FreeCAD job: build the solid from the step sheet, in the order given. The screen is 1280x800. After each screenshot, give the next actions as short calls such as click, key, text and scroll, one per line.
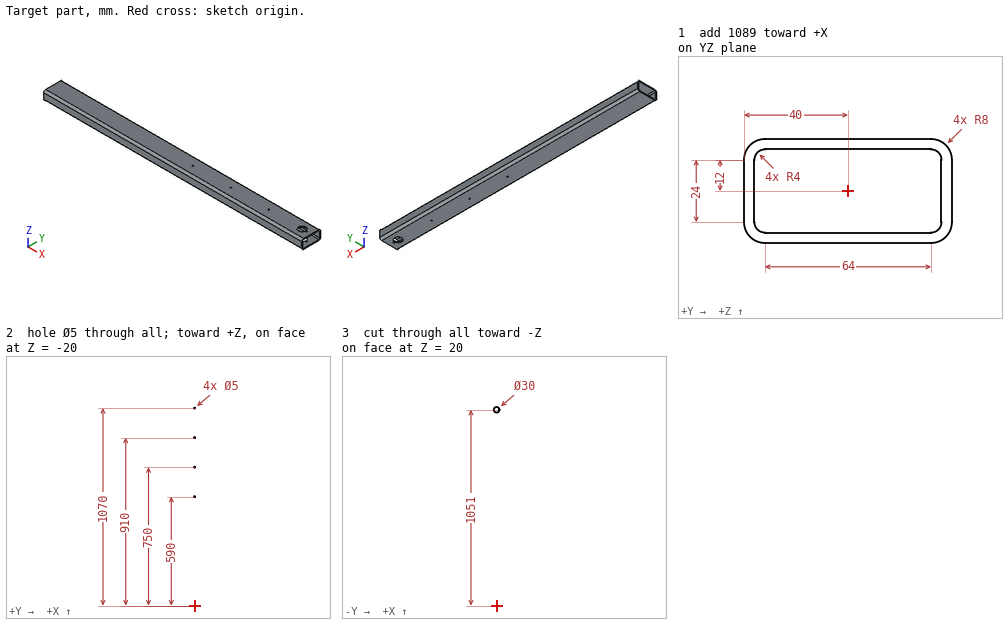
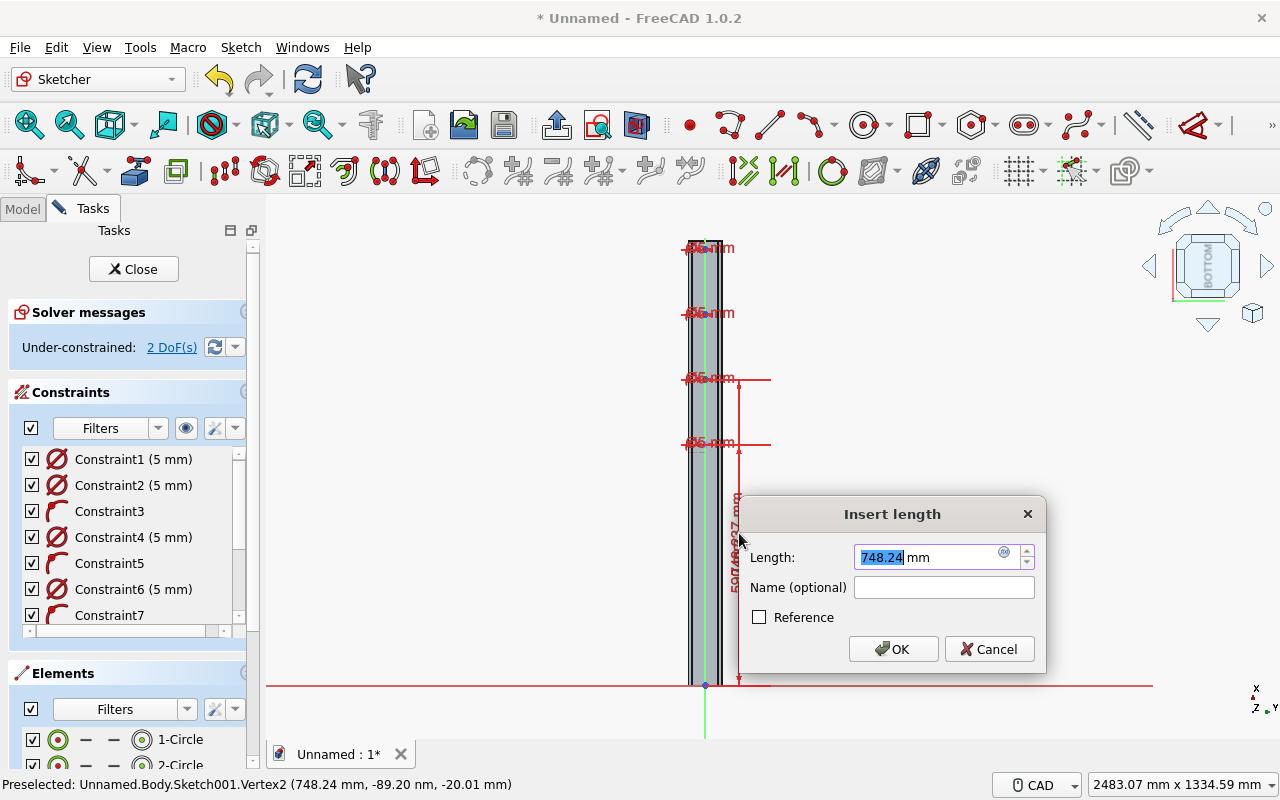
text(750)
key(Return)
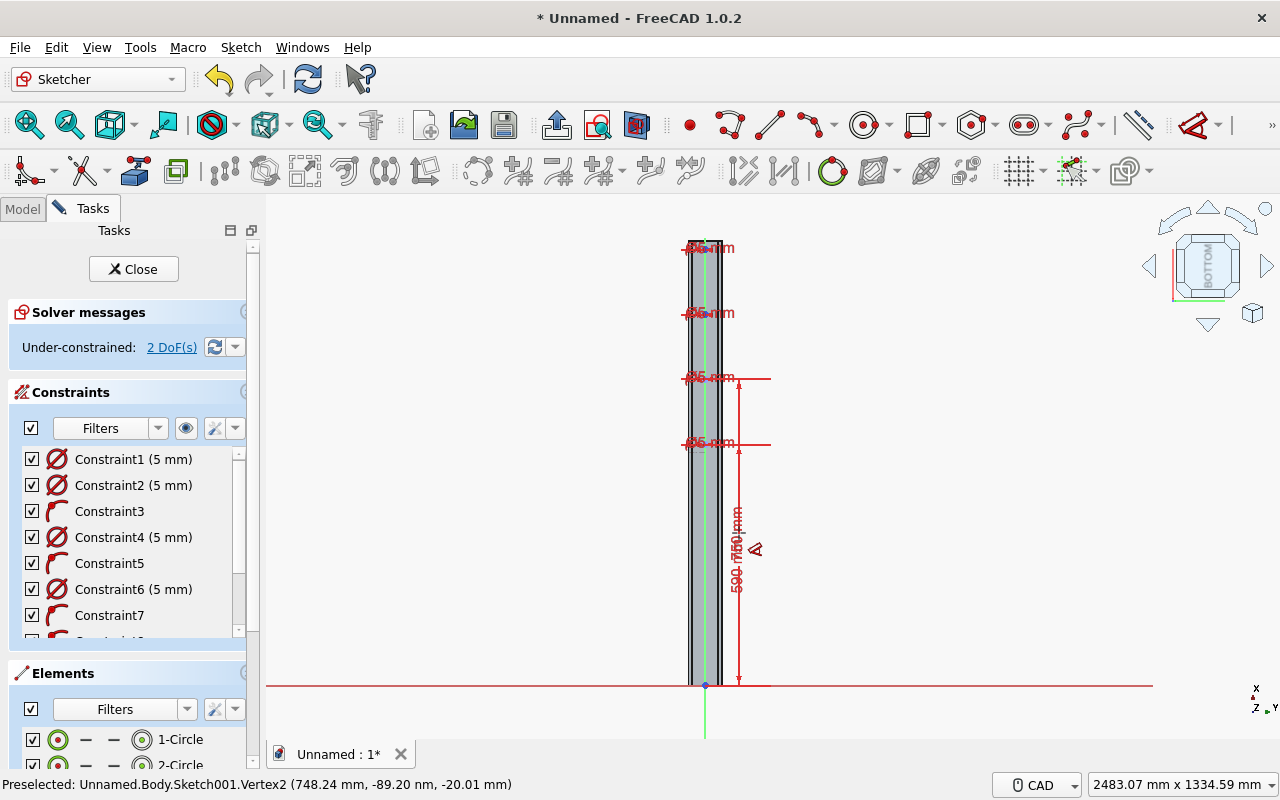
click(705, 315)
click(739, 500)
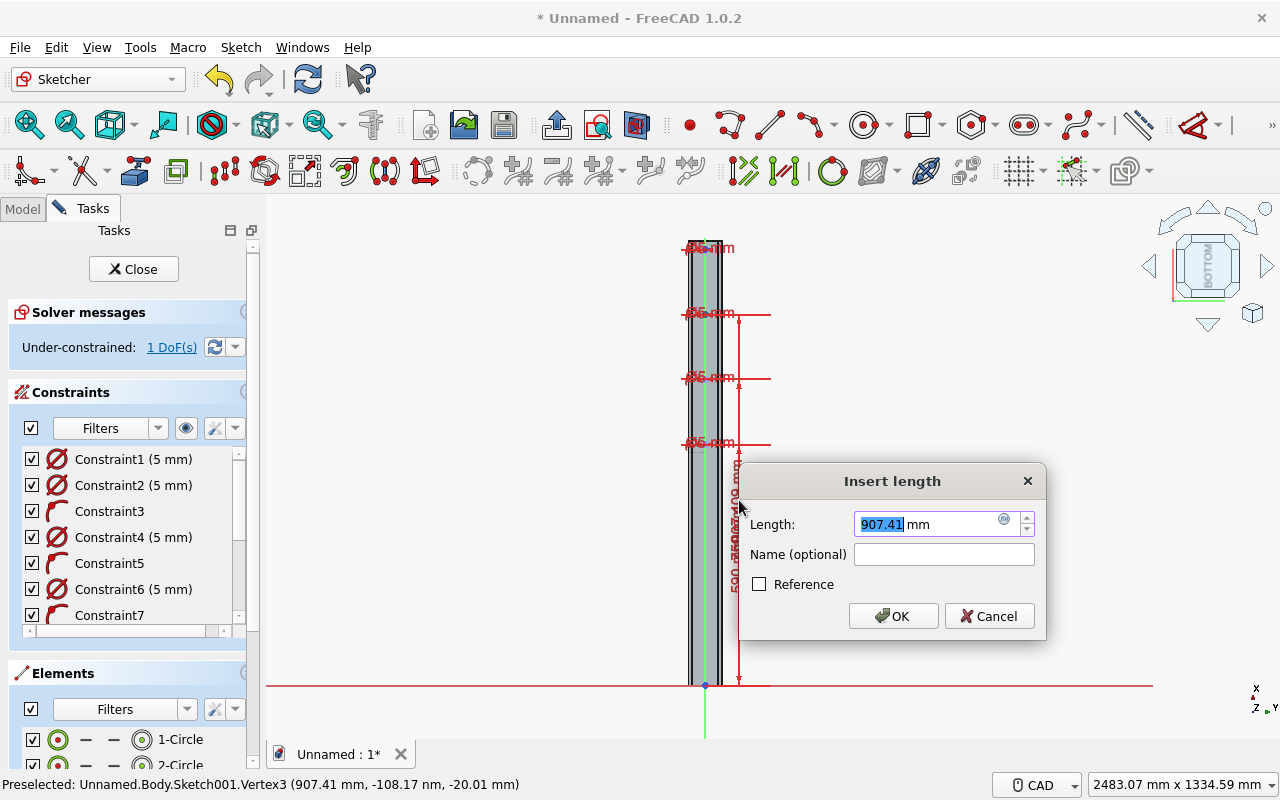
text(910)
key(Return)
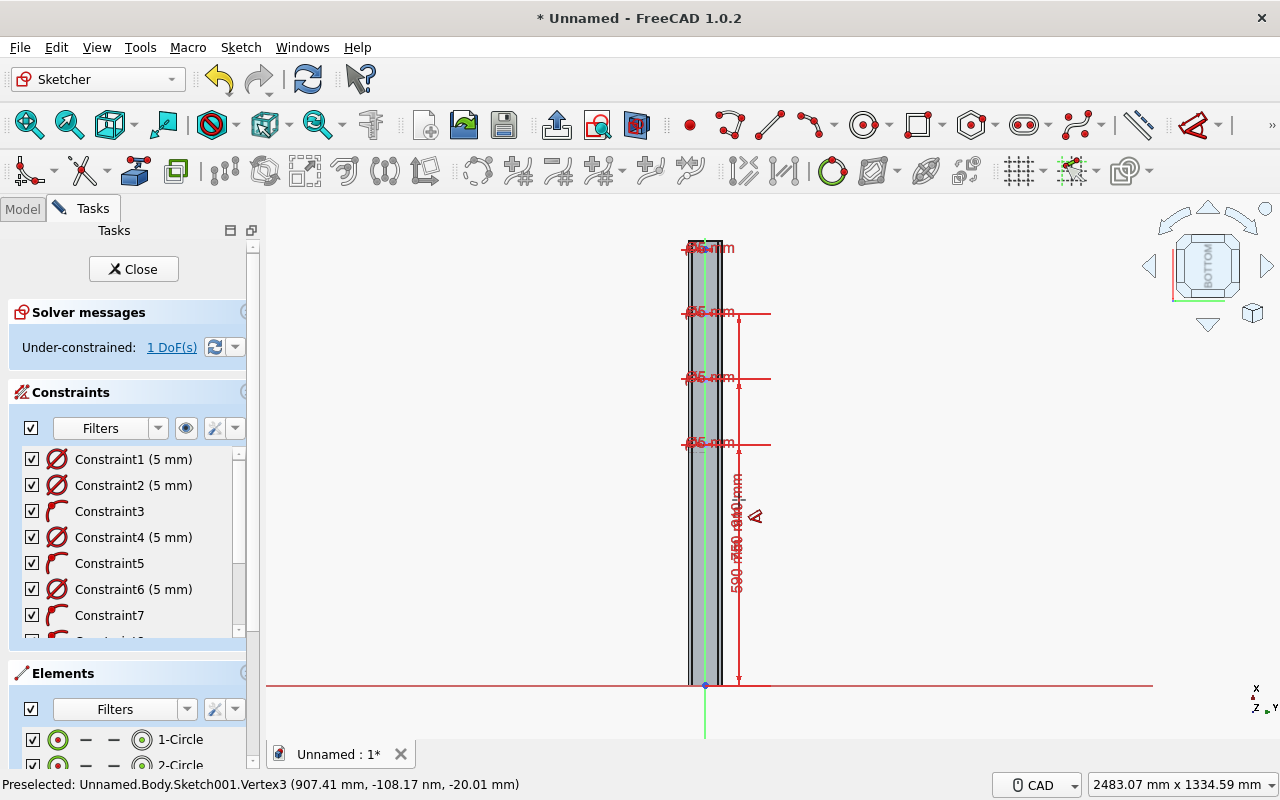
click(705, 250)
click(739, 468)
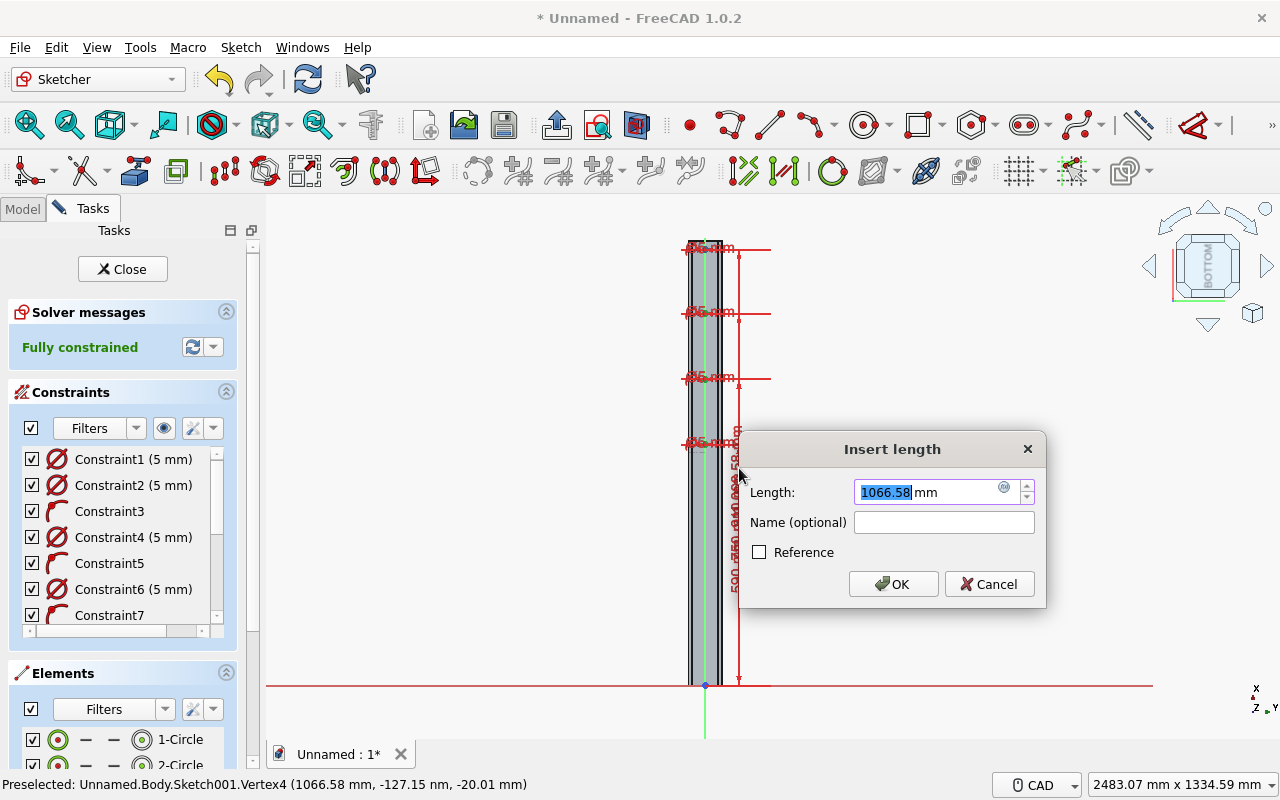
text(1070)
key(Return)
key(Escape)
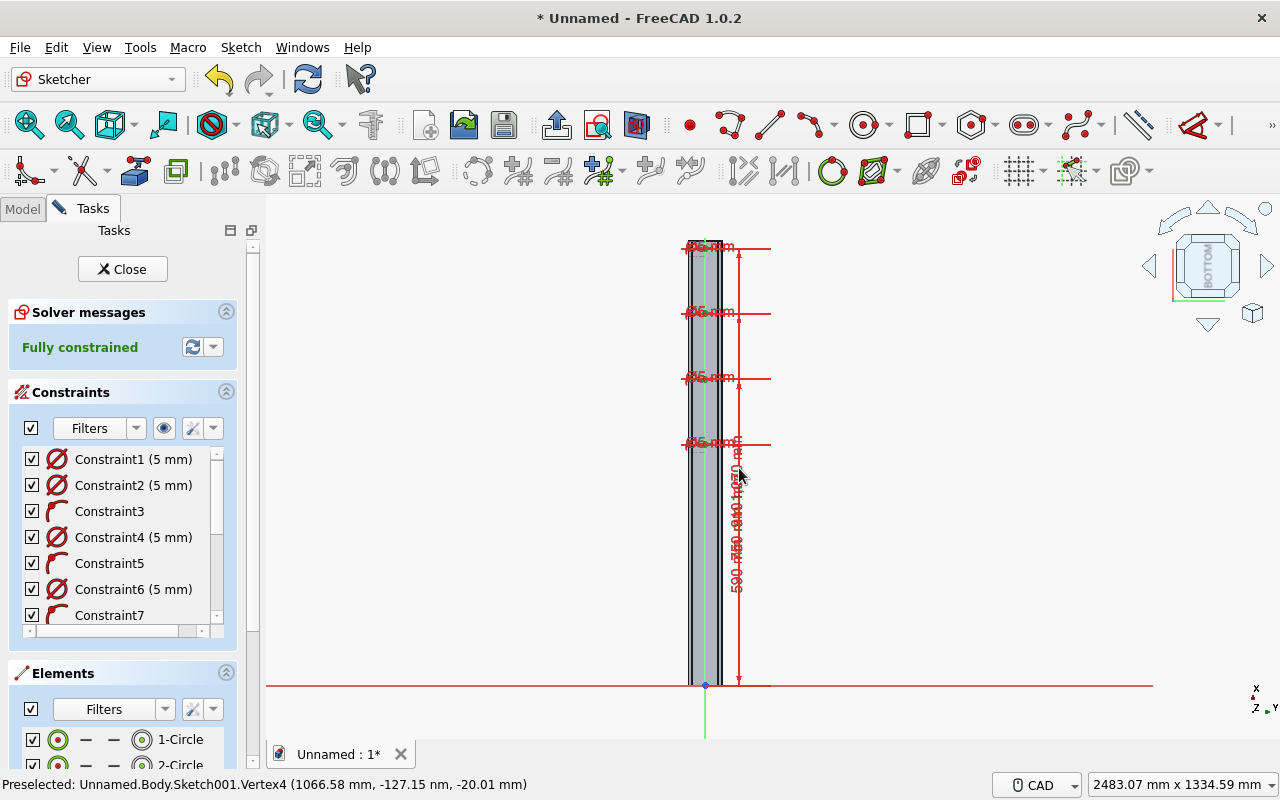
click(123, 269)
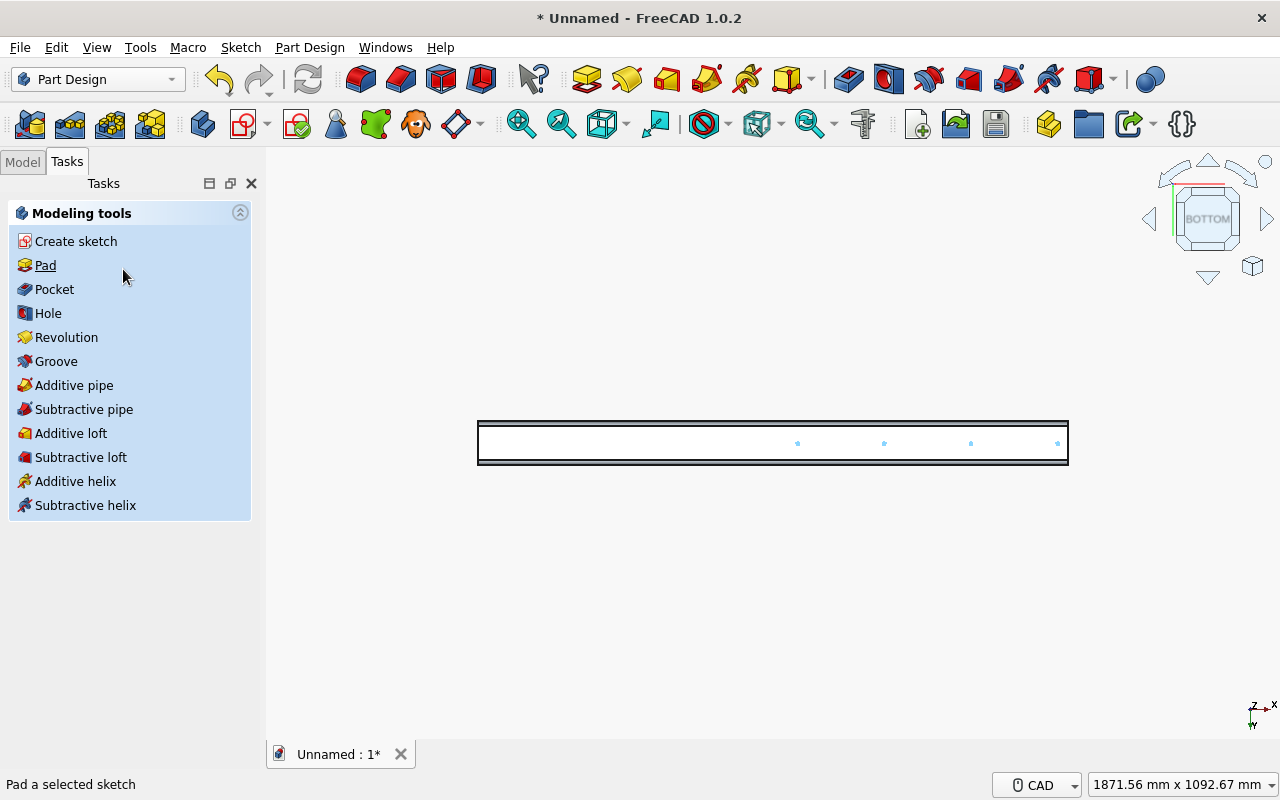
click(890, 80)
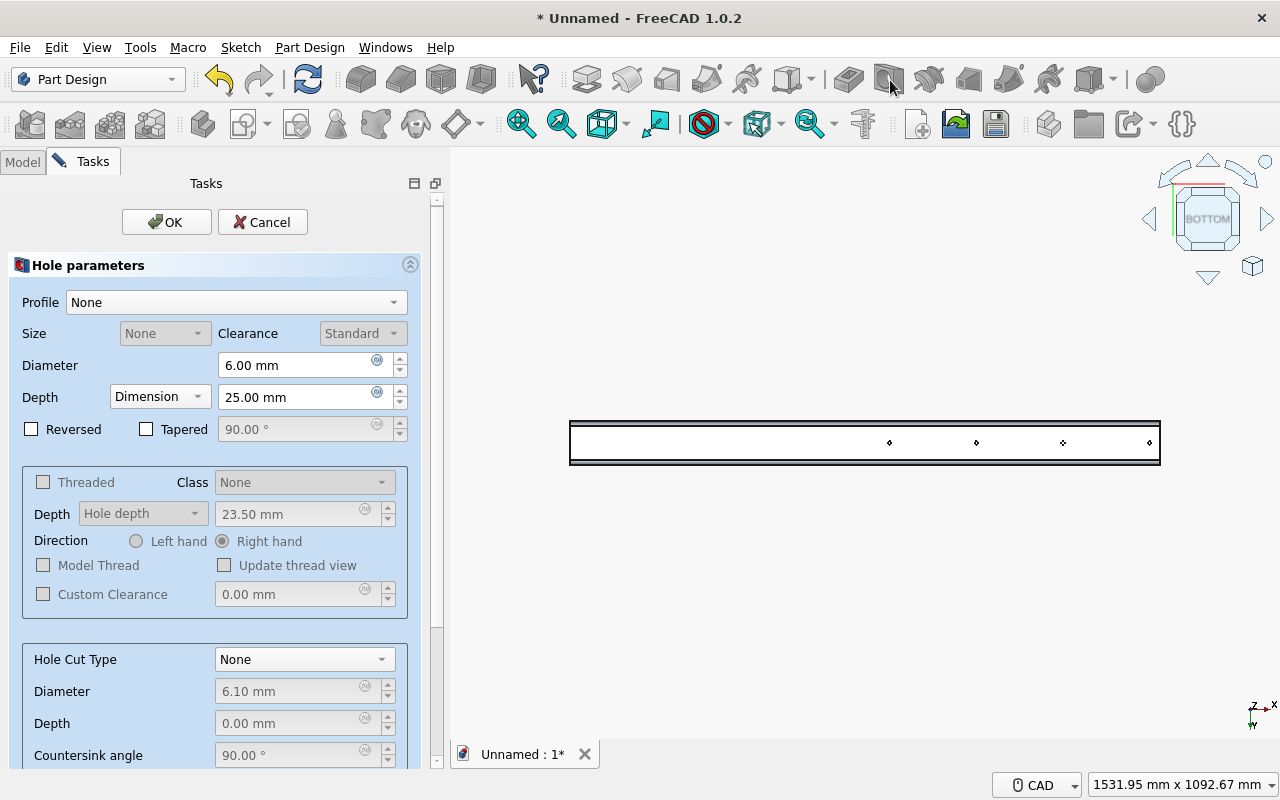
triple_click(305, 365)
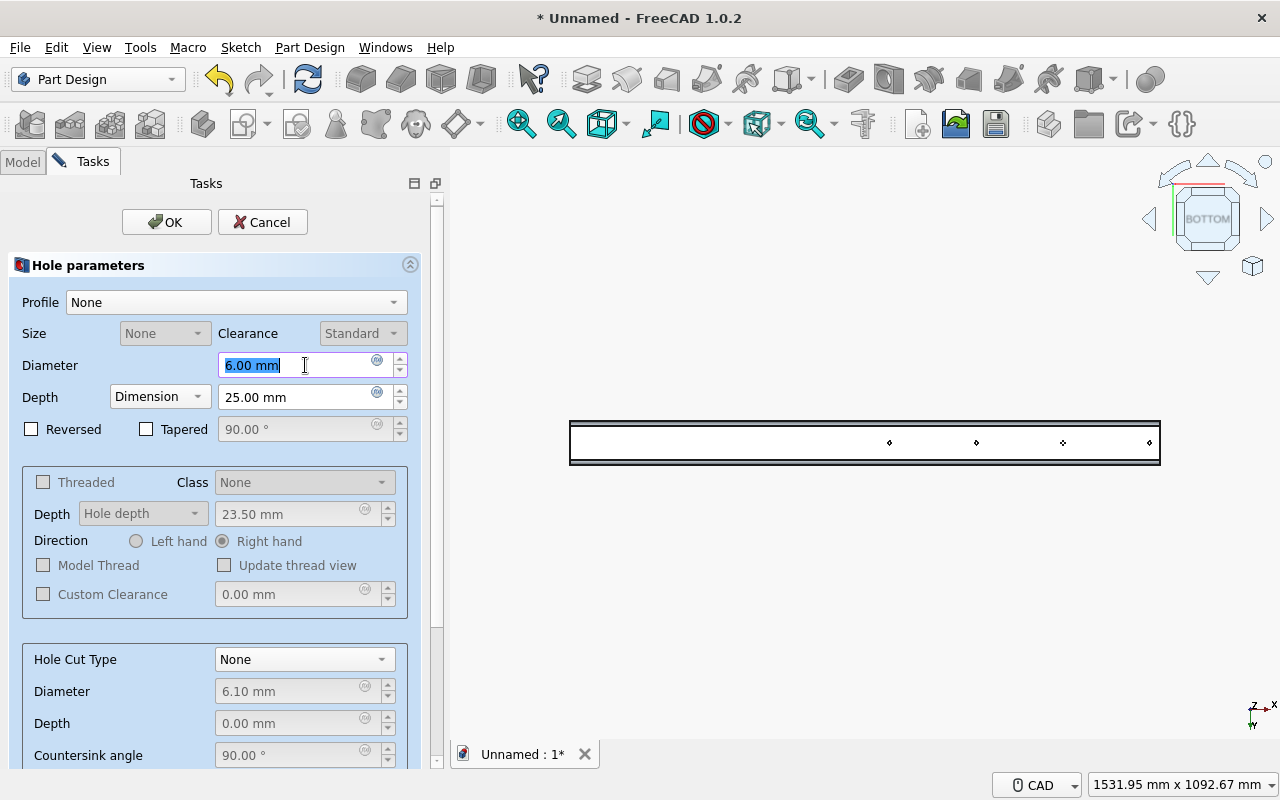
text(5)
key(Tab)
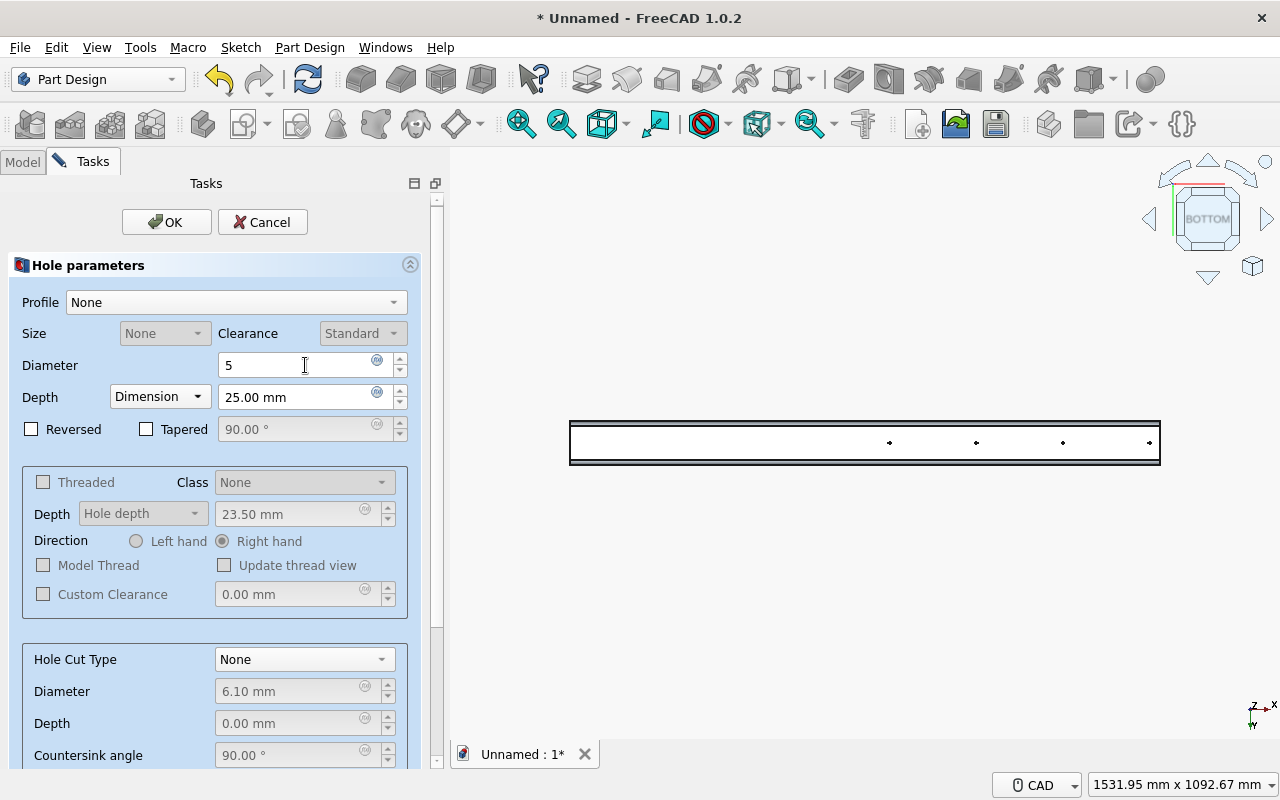
click(161, 396)